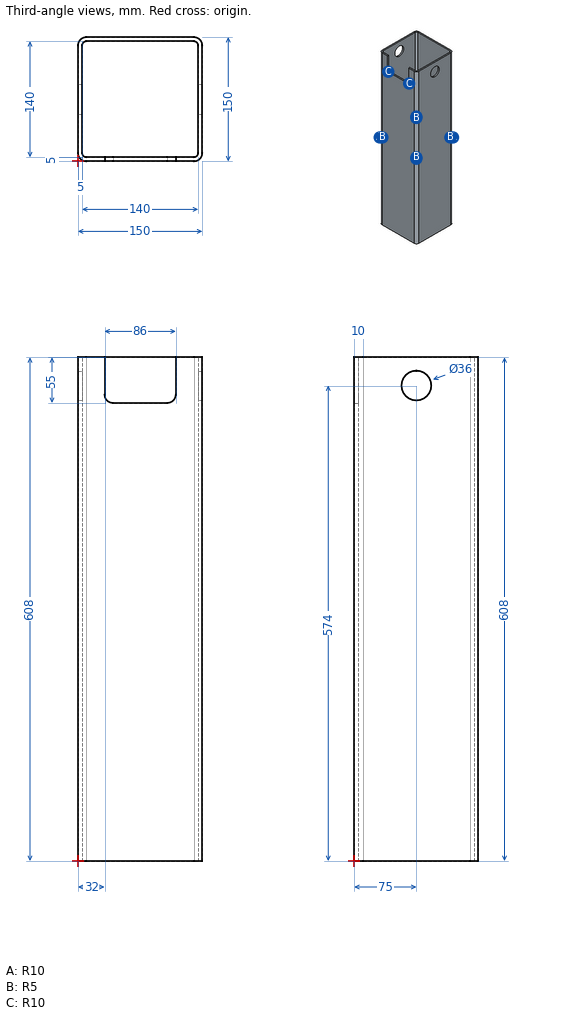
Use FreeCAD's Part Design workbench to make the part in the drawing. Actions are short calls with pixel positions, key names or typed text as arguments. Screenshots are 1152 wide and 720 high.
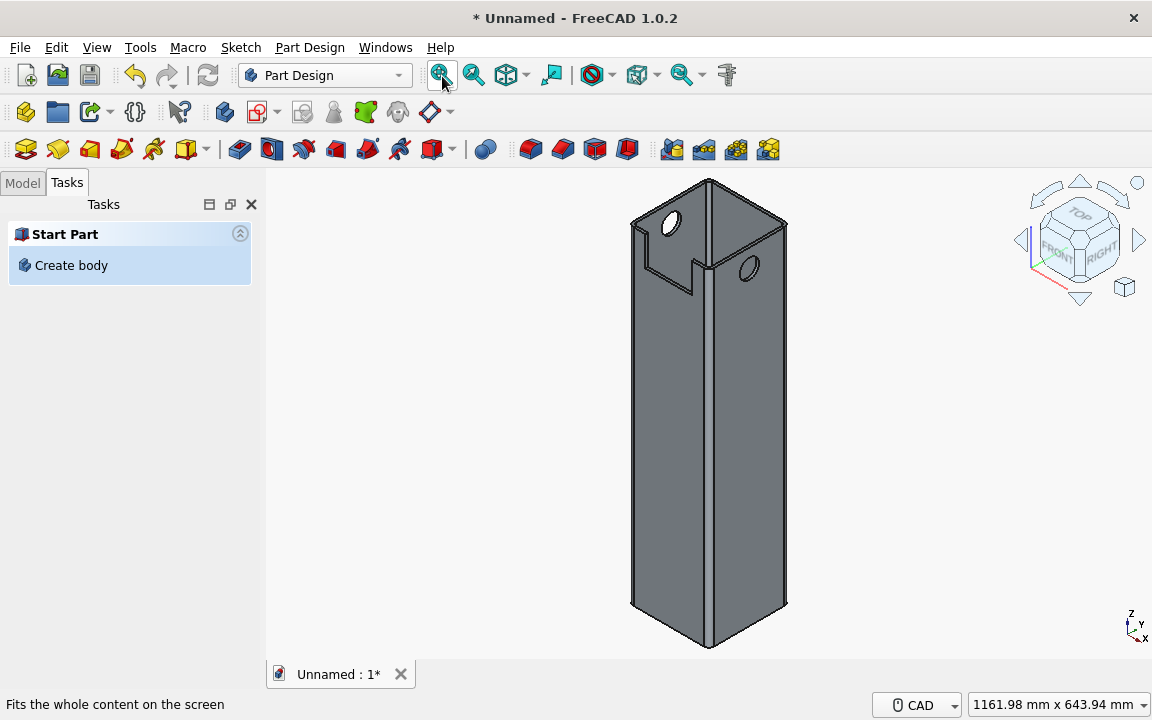
scroll(647, 267, up, 12)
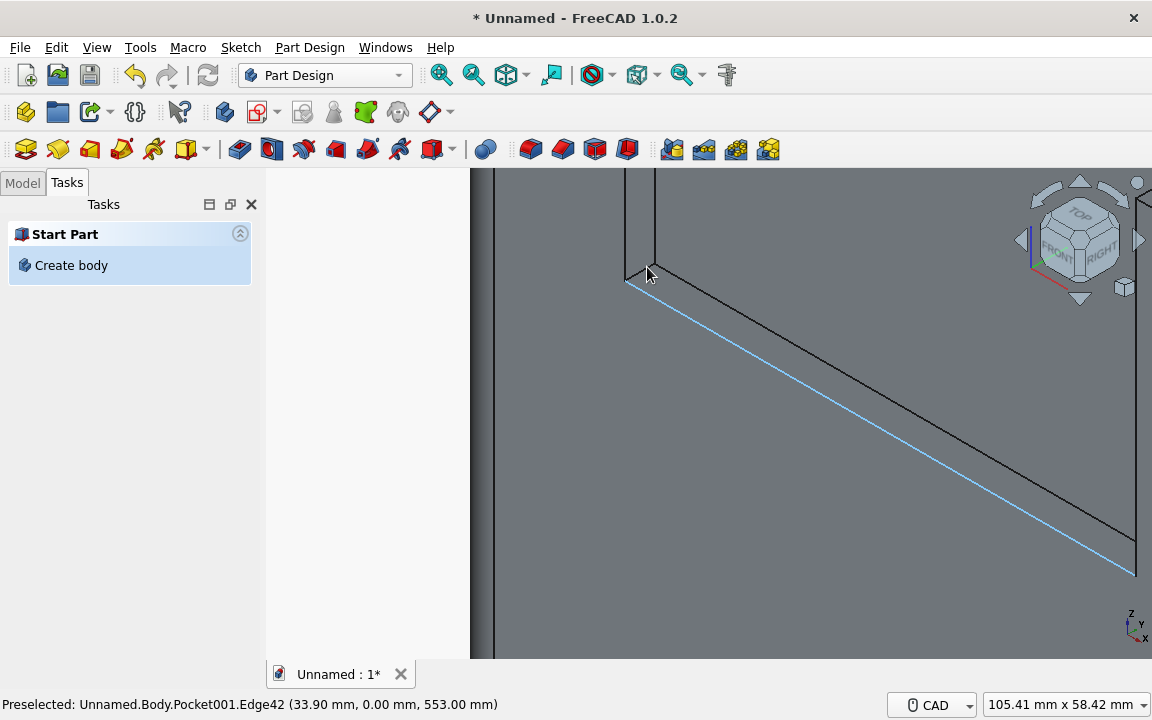
key(v)
key(f)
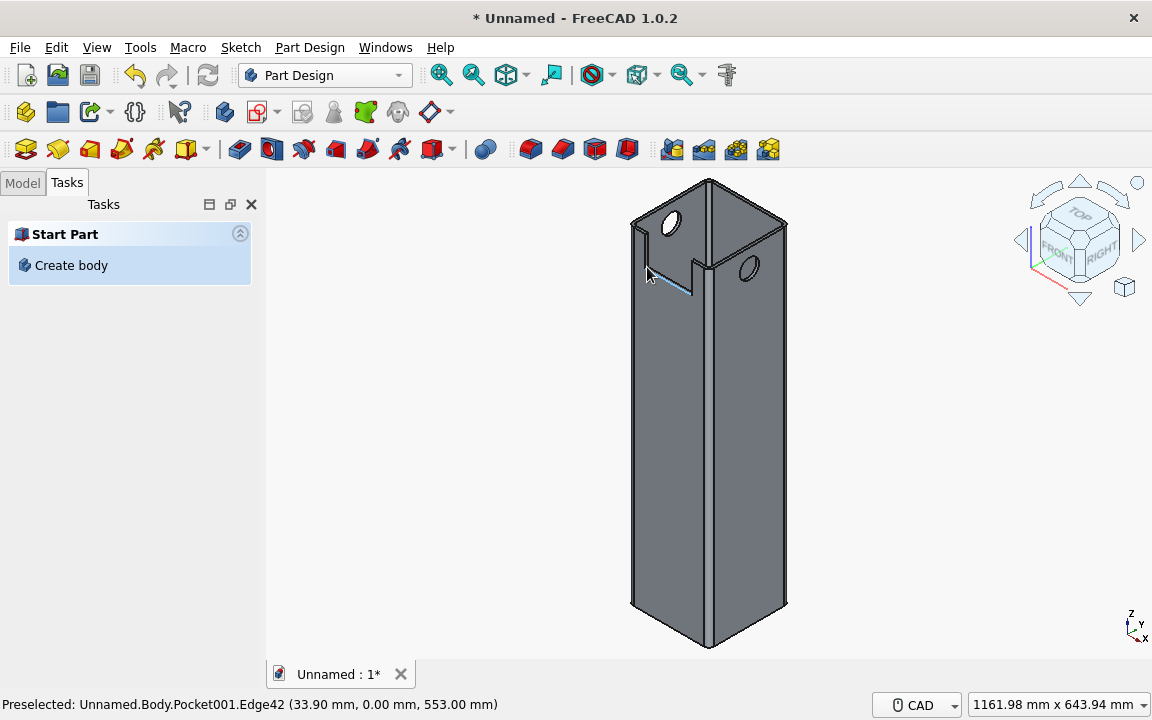
key(1)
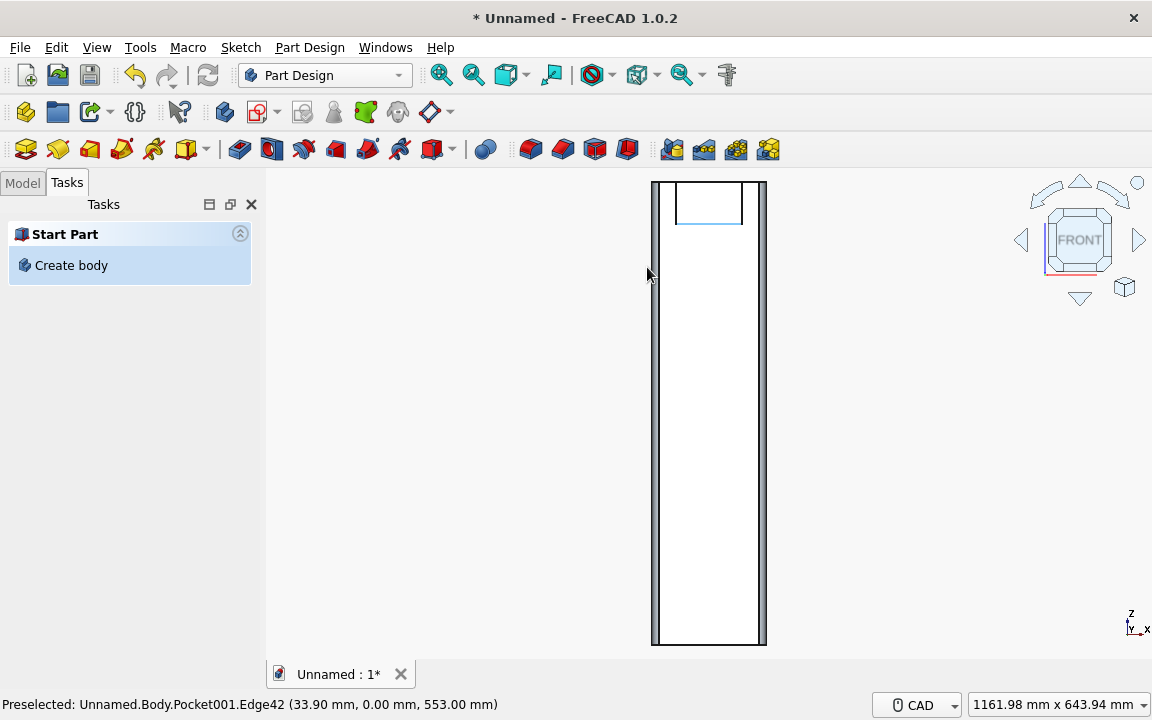
scroll(676, 223, up, 12)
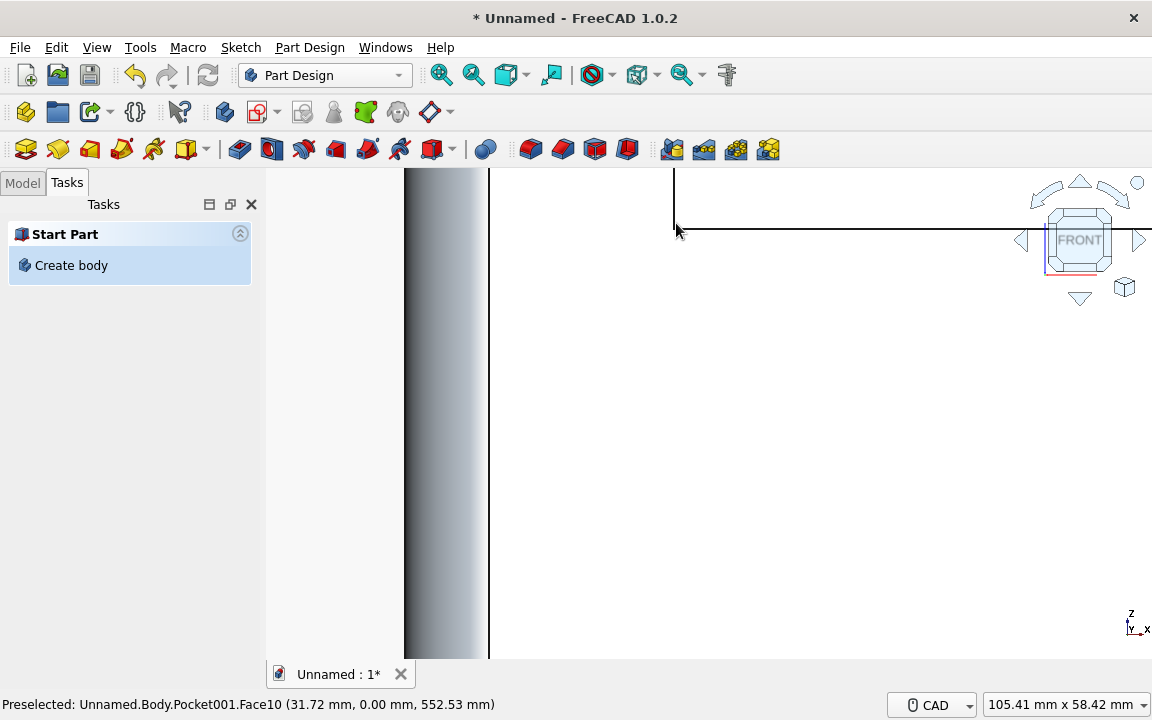
key(v)
key(f)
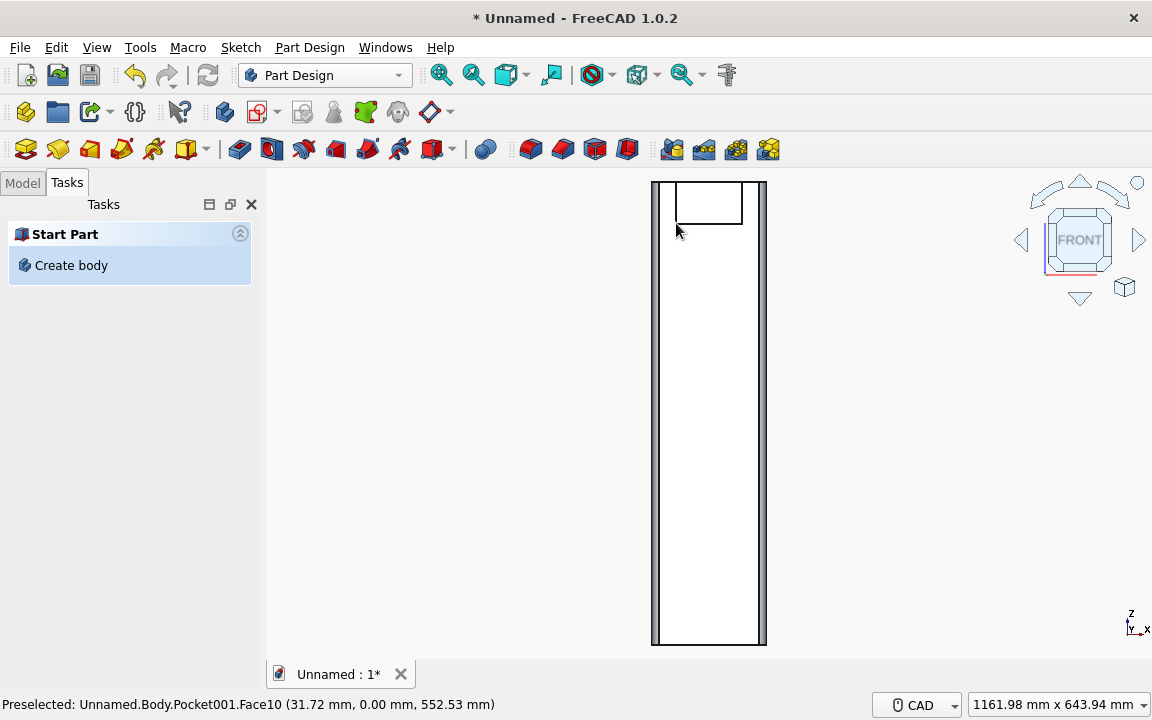
key(3)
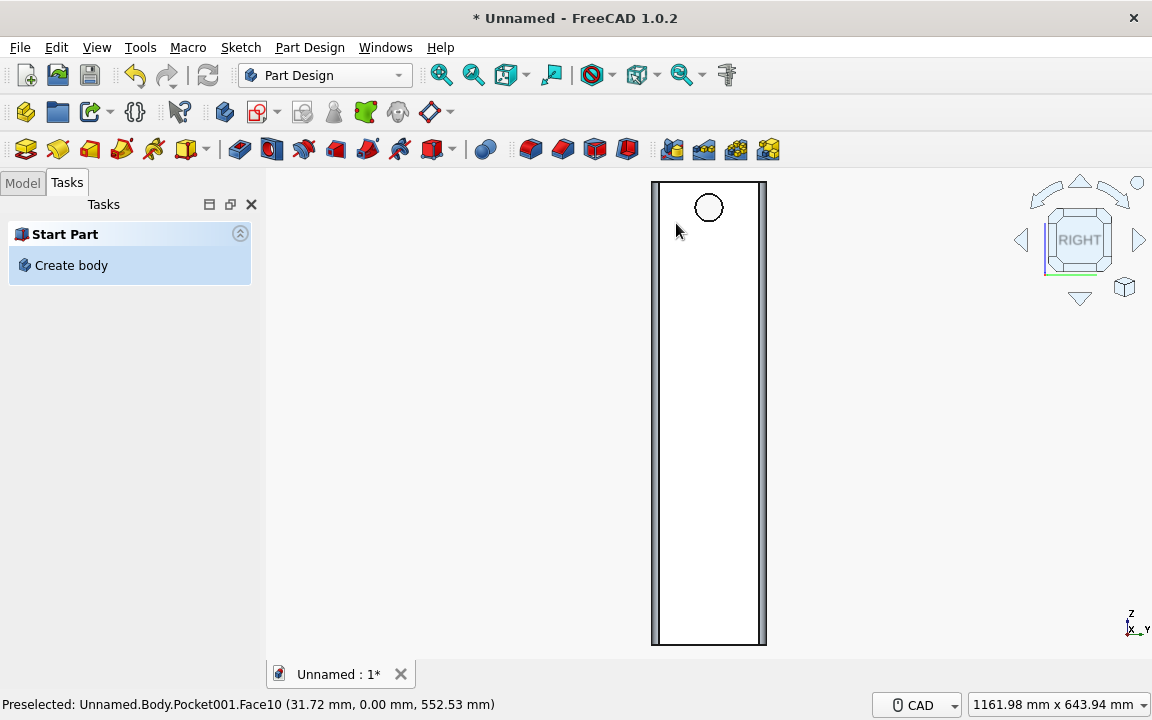
scroll(654, 223, up, 12)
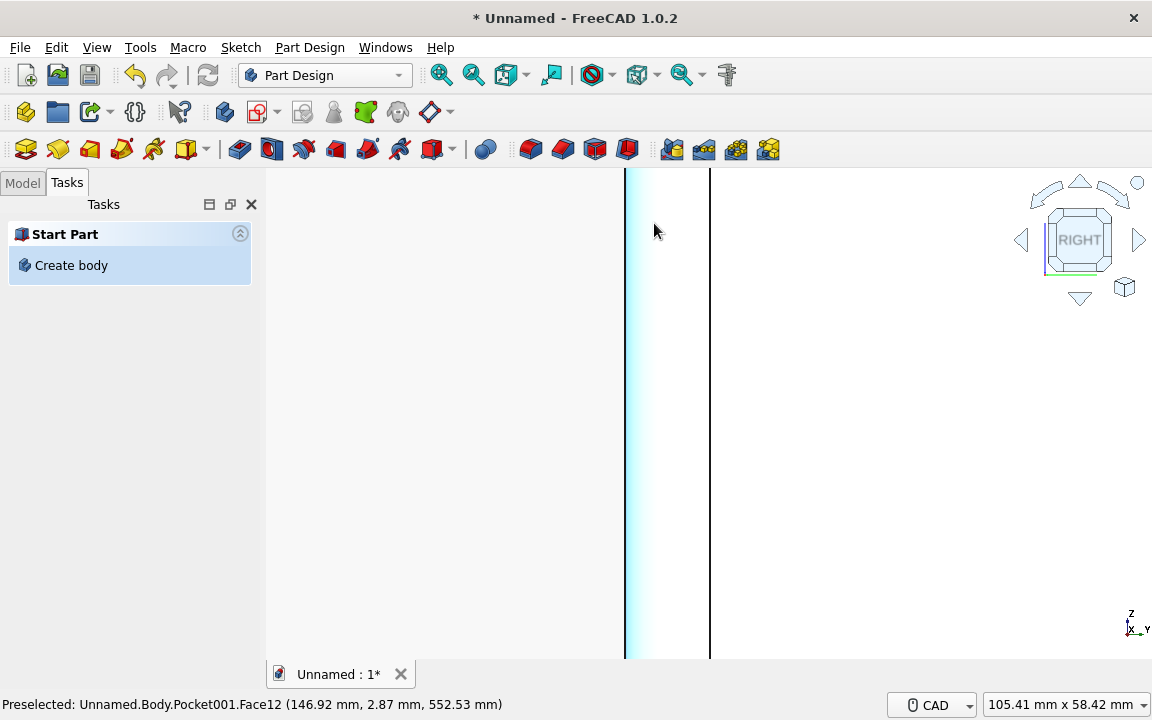
key(v)
key(f)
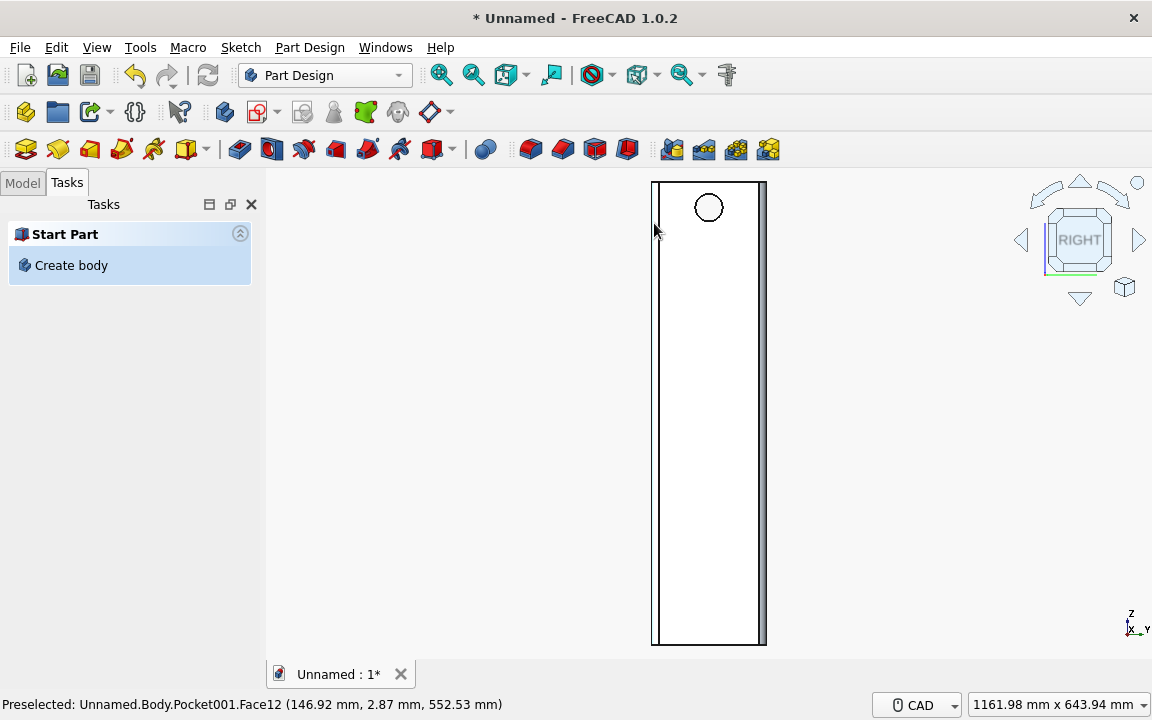
key(5)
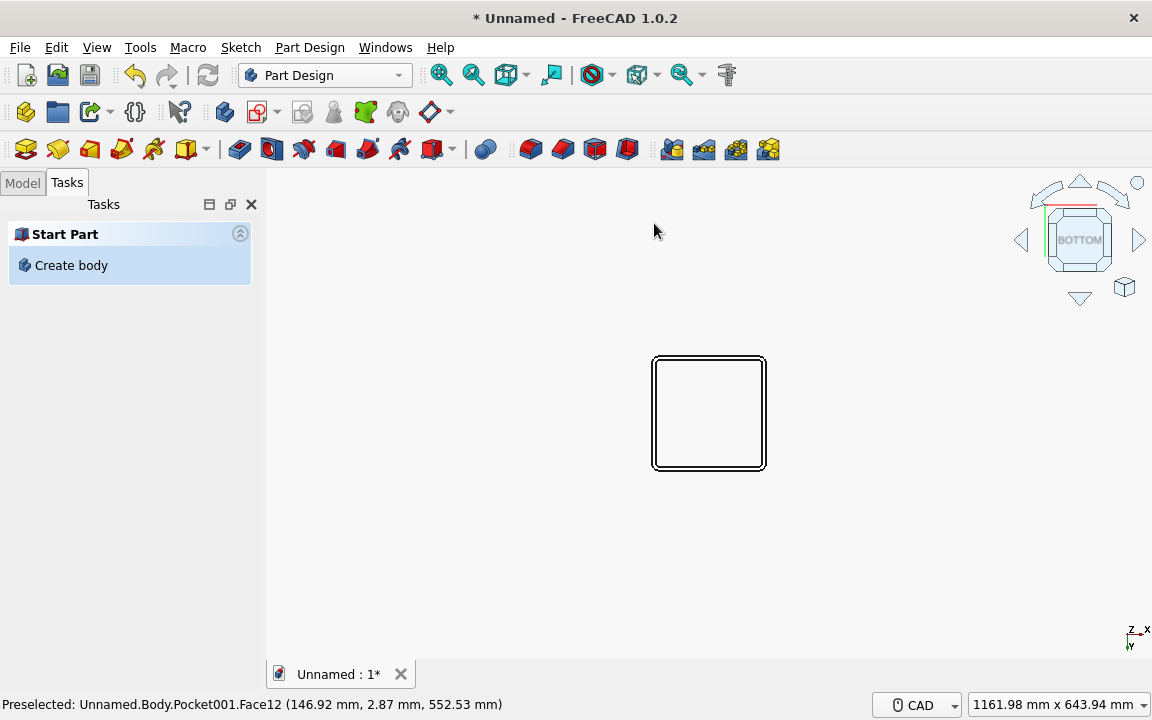
key(v)
key(f)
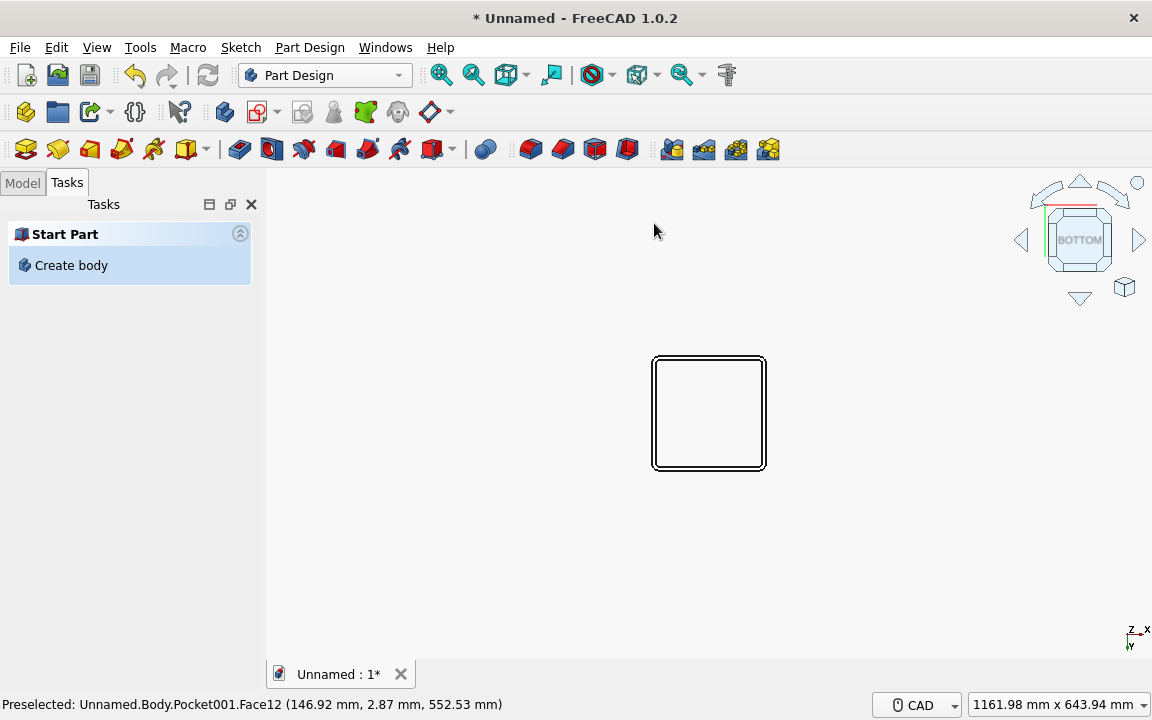
scroll(676, 357, up, 12)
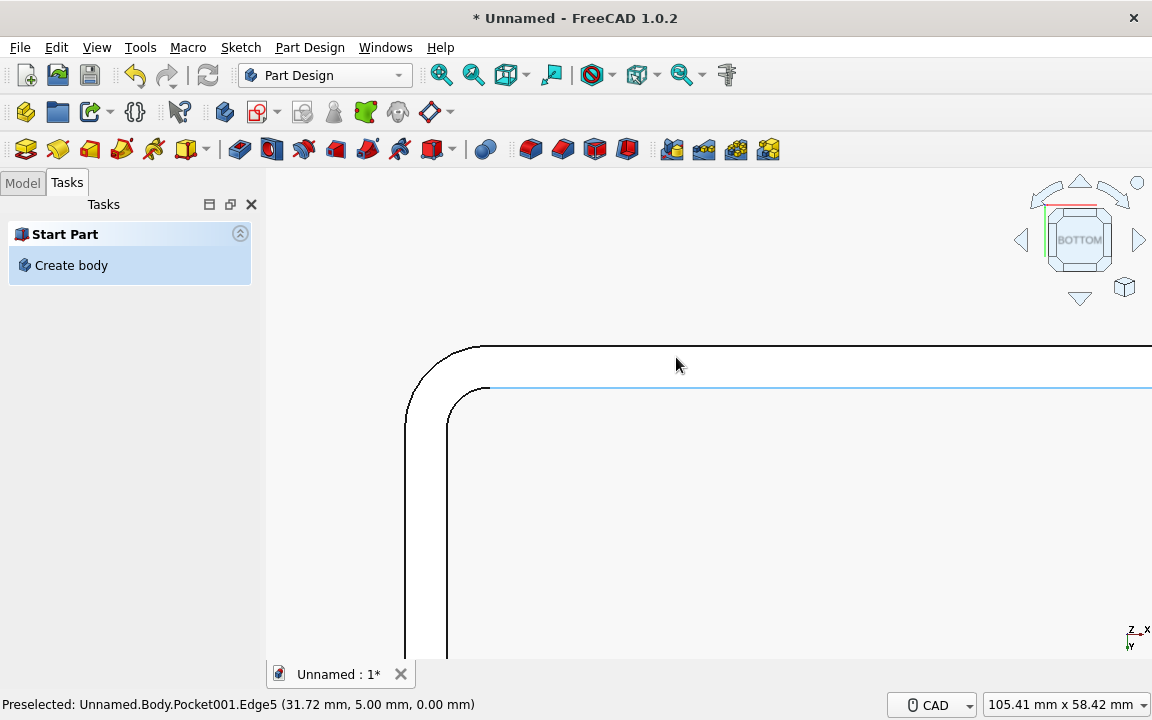
key(v)
key(f)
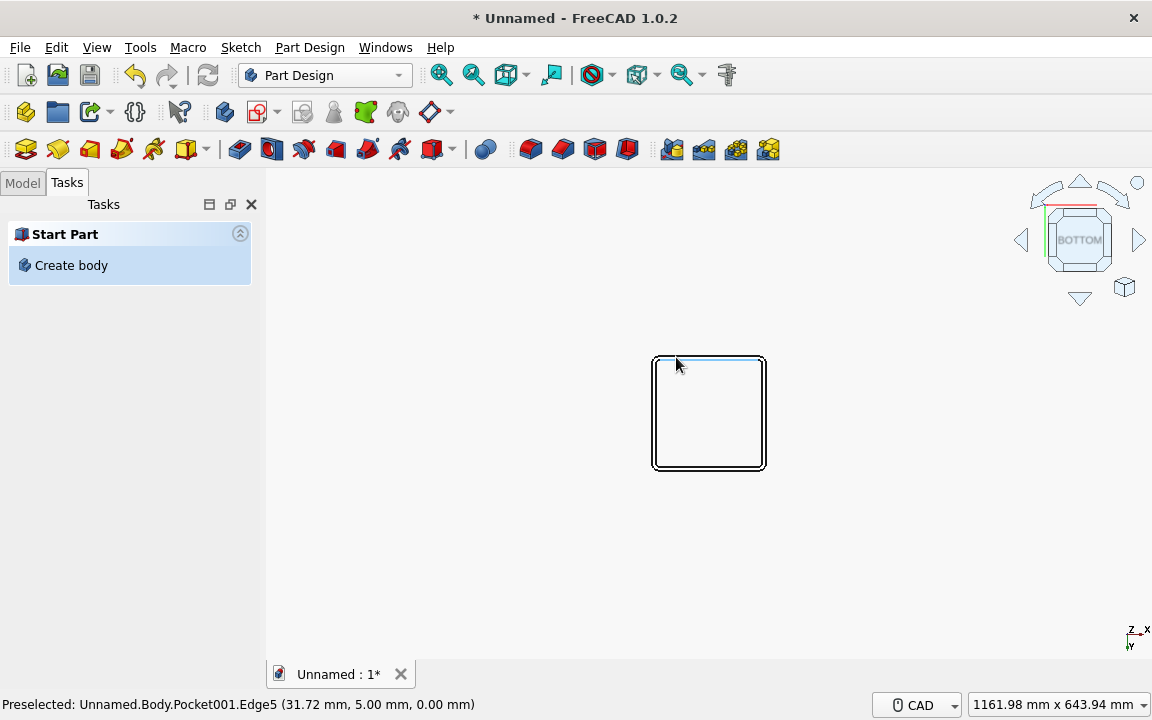
key(4)